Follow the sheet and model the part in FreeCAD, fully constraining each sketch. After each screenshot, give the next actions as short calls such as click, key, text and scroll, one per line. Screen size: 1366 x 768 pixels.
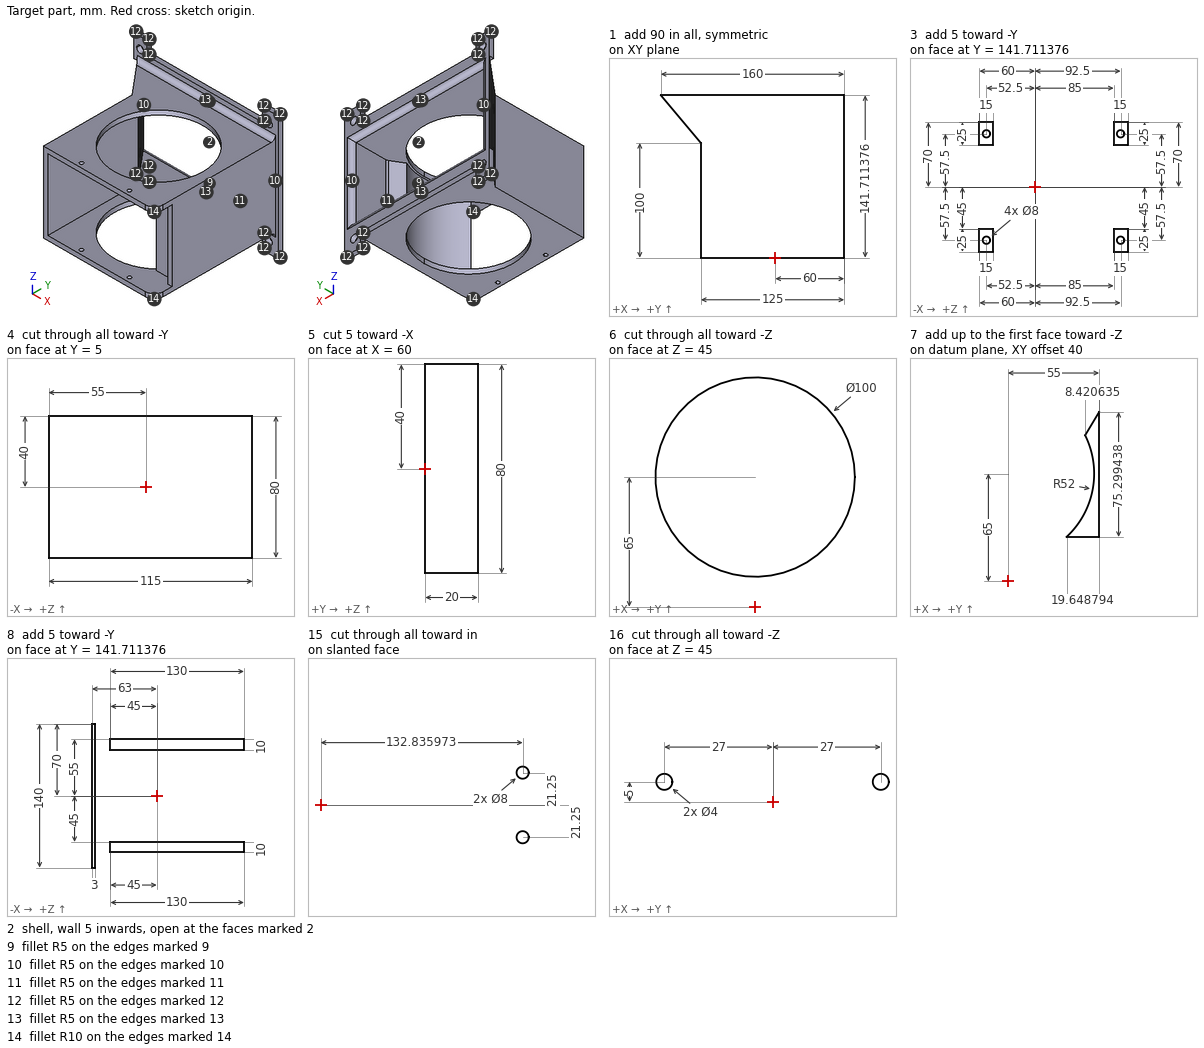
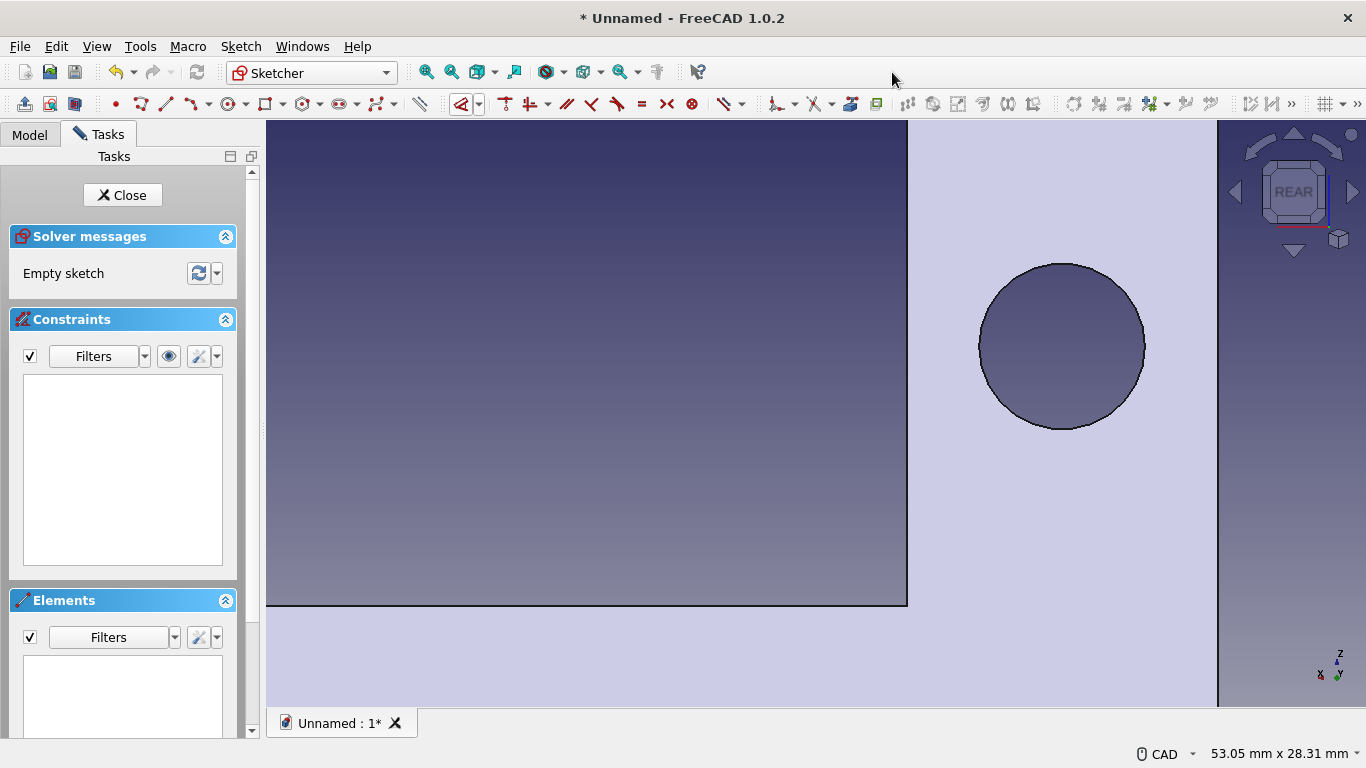
scroll(963, 237, down, 10)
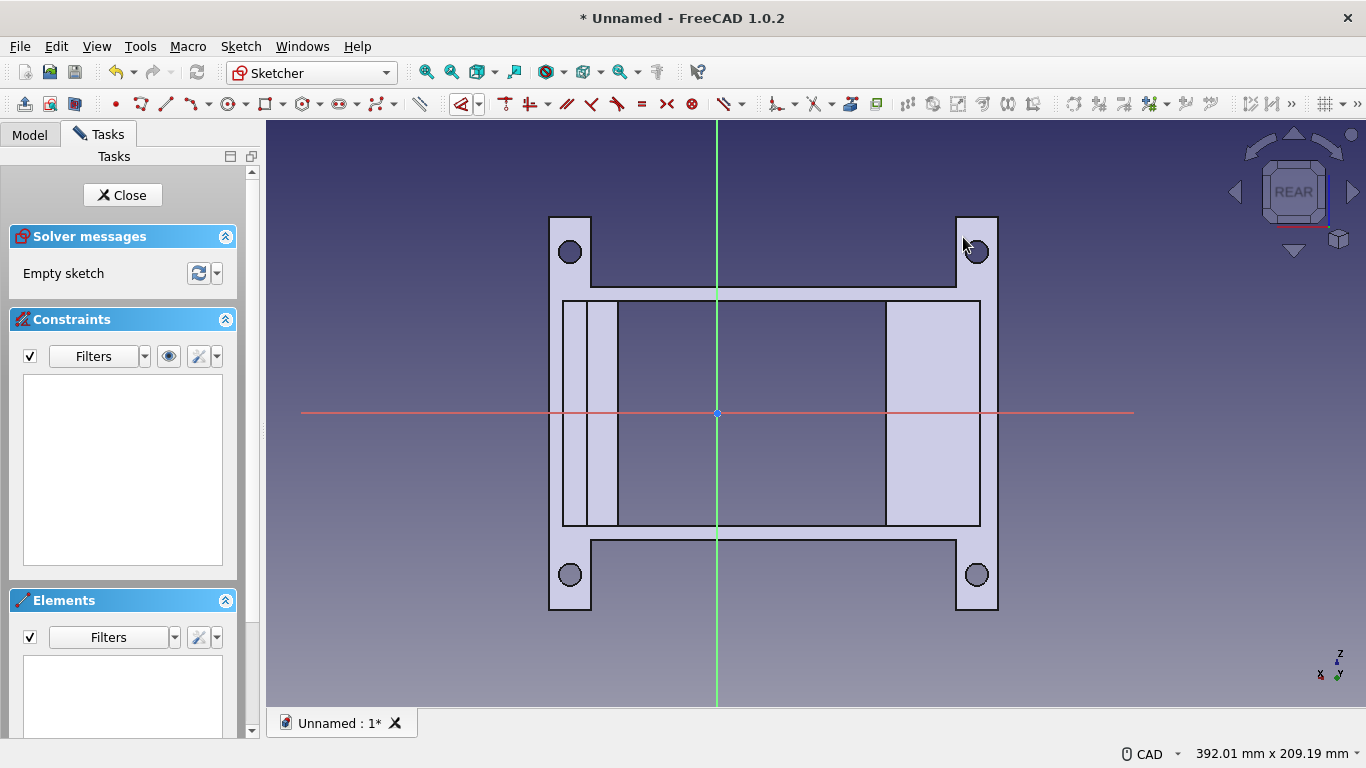
click(264, 104)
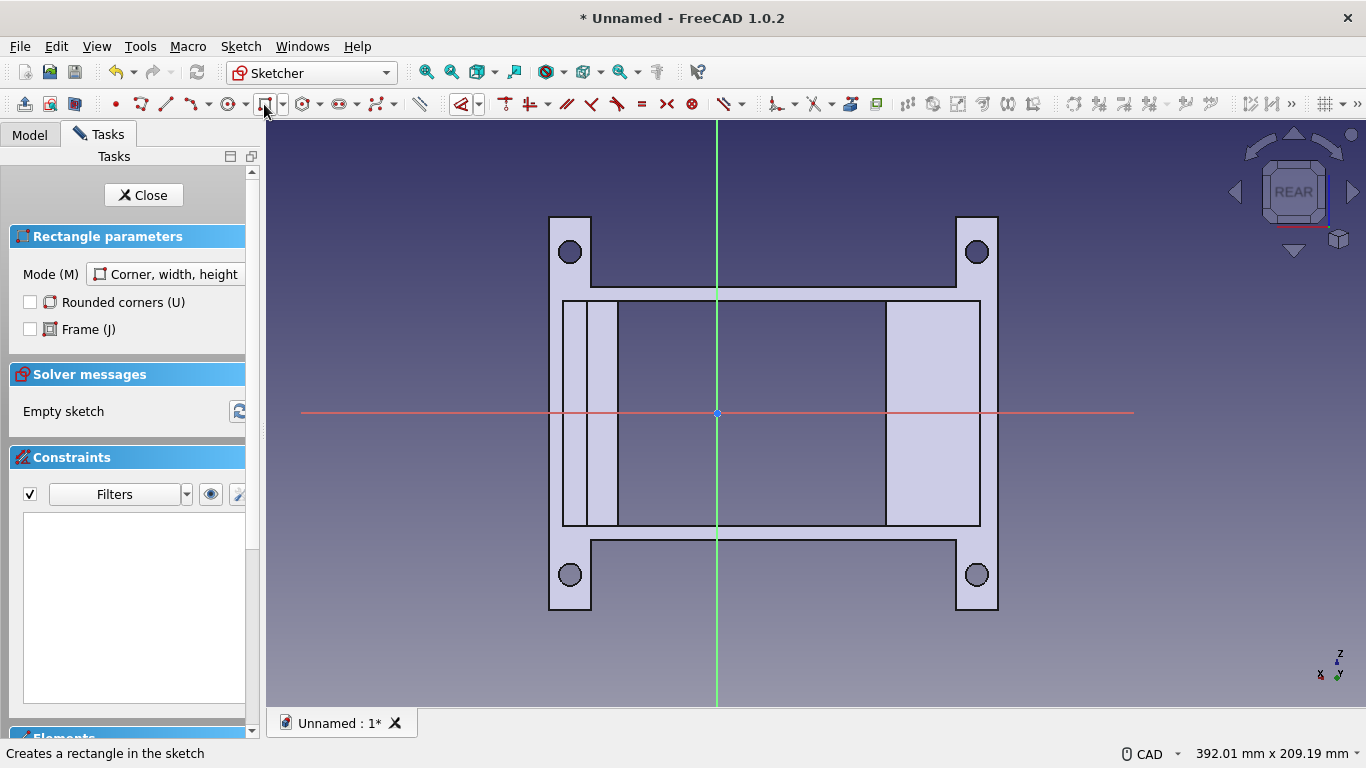
click(591, 540)
move(956, 568)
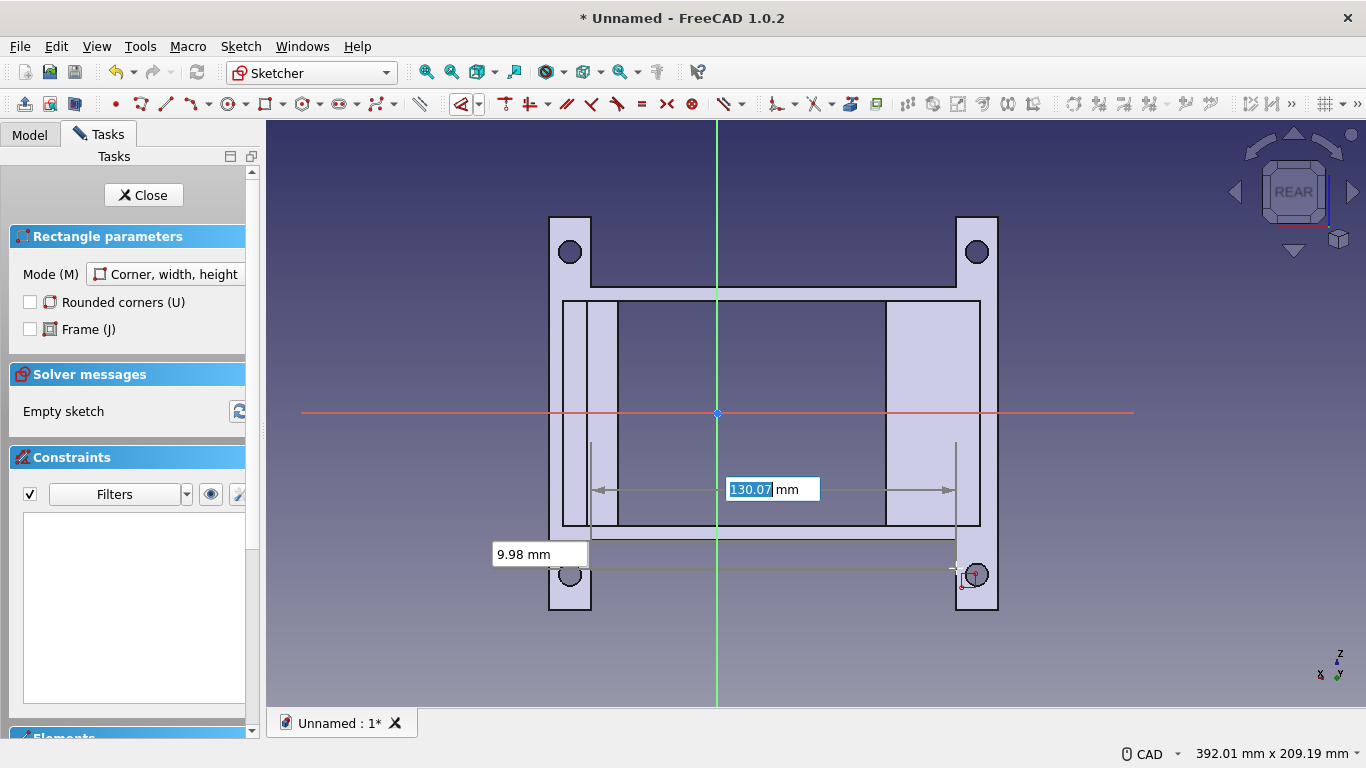
text(130)
key(Tab)
text(10)
key(Return)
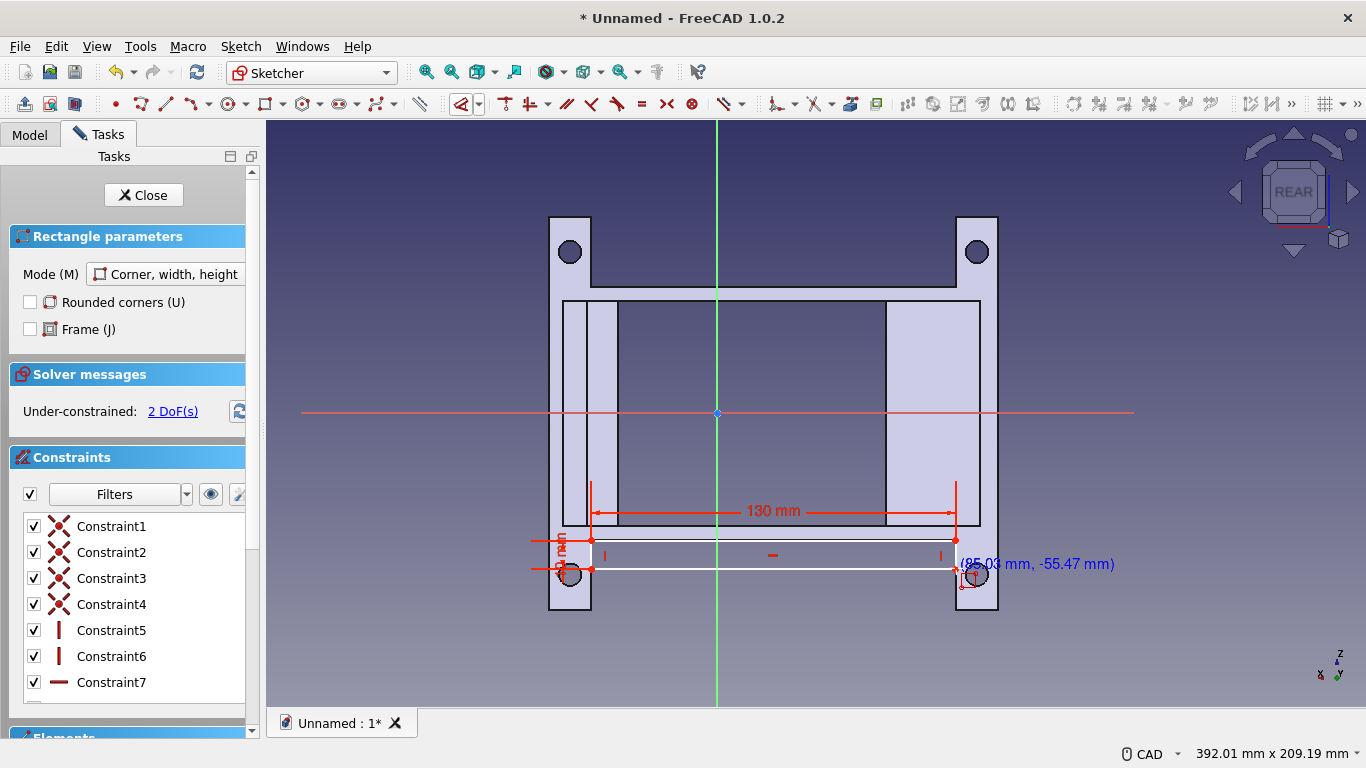
click(591, 259)
move(956, 287)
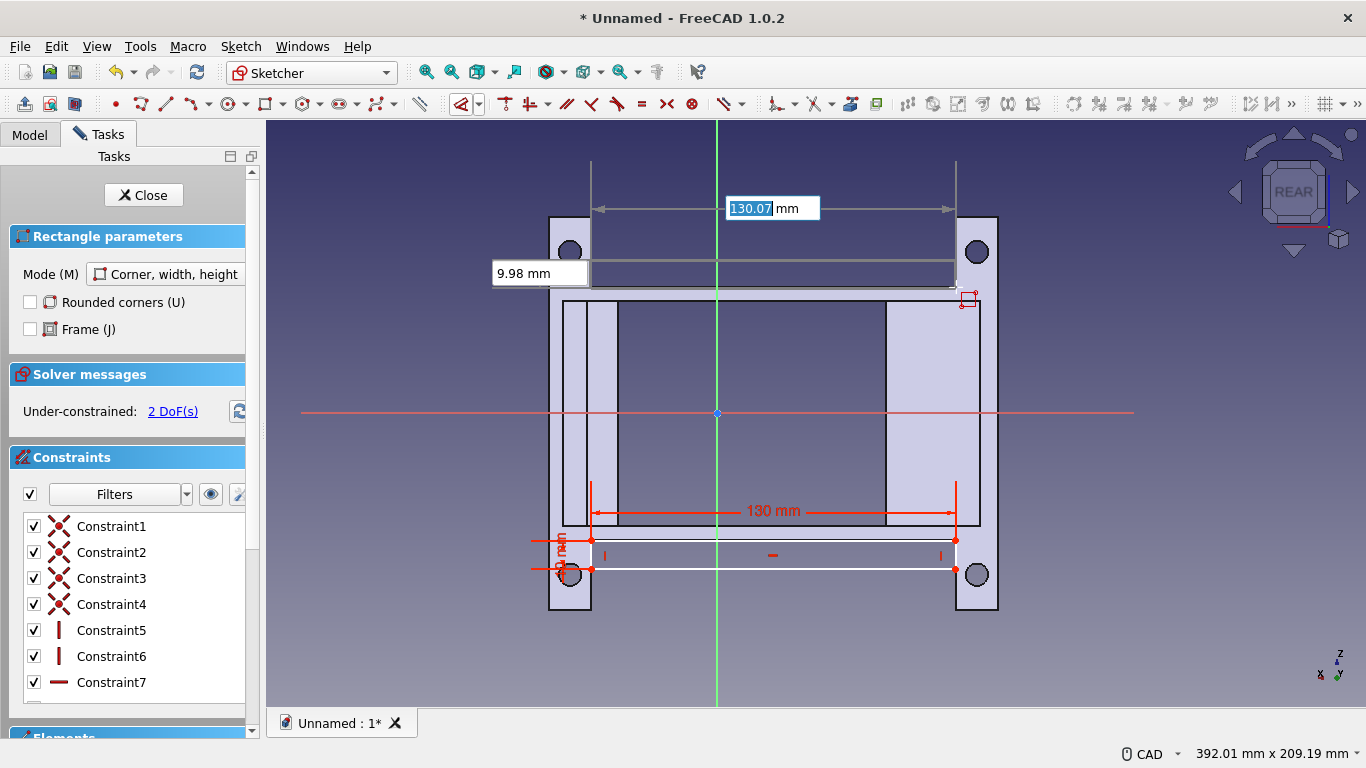
text(130)
key(Tab)
text(10)
key(Return)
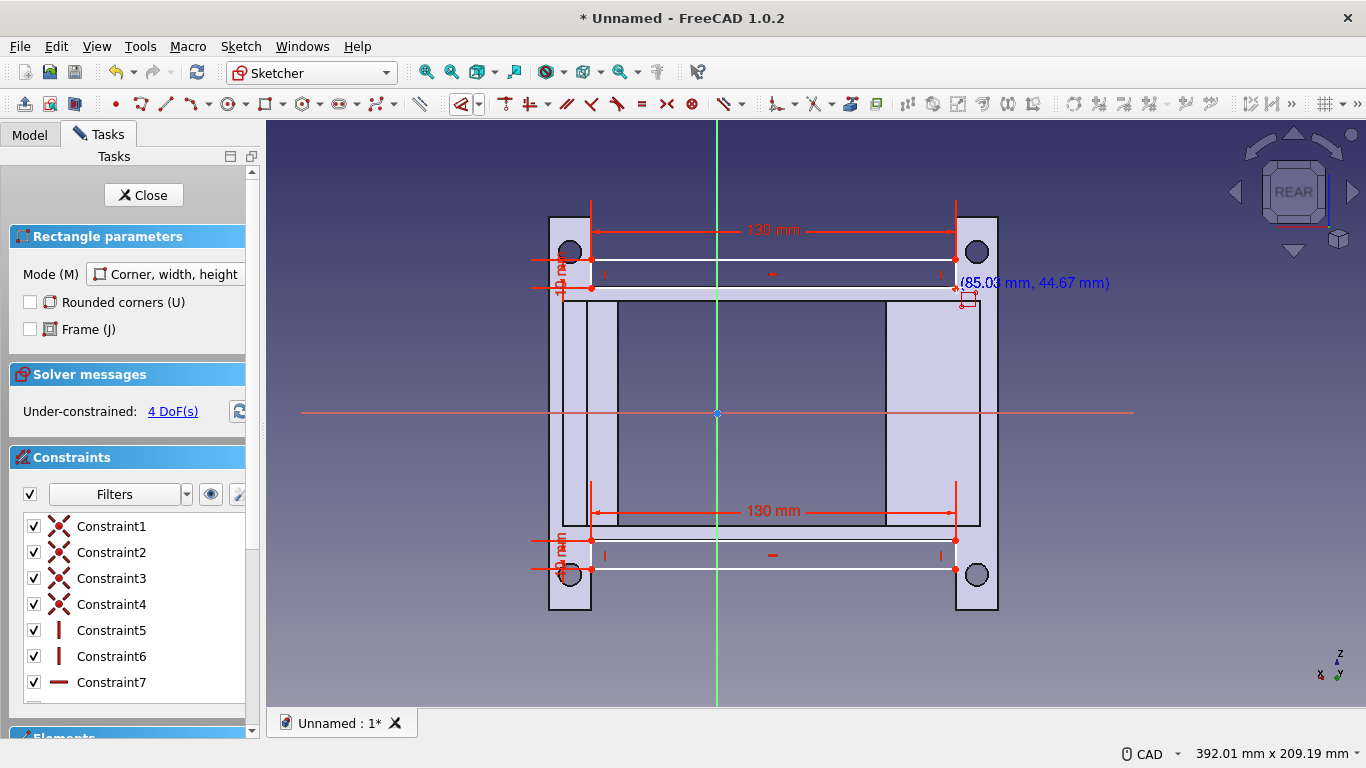
scroll(541, 217, up, 4)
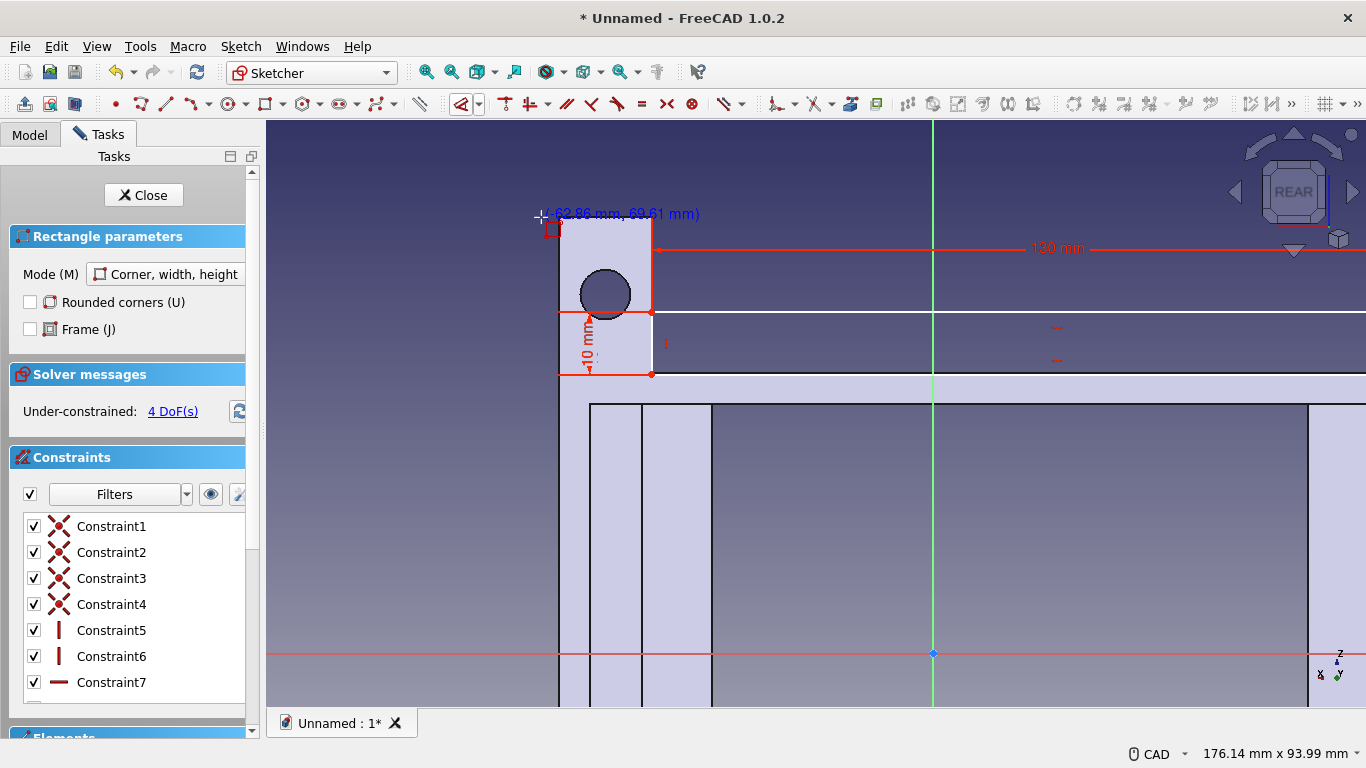
click(540, 217)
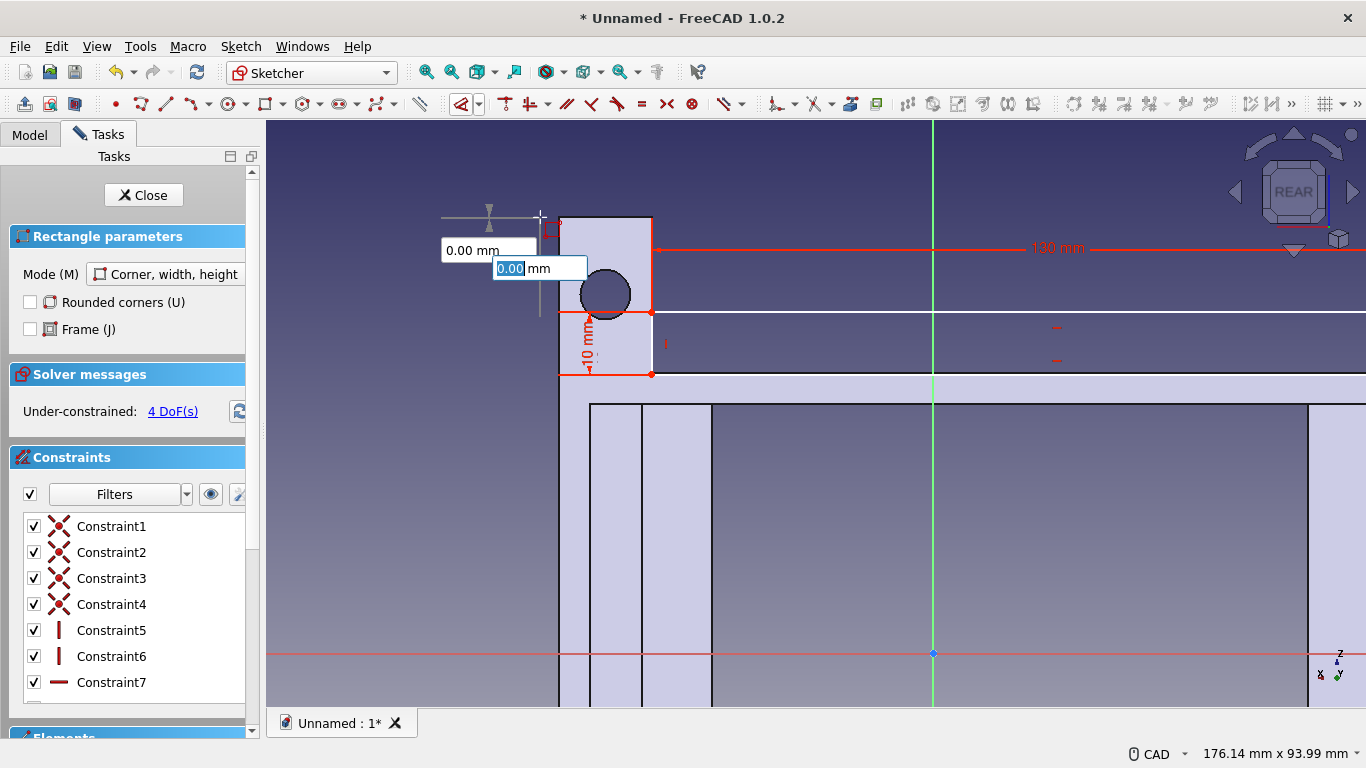
scroll(540, 217, down, 4)